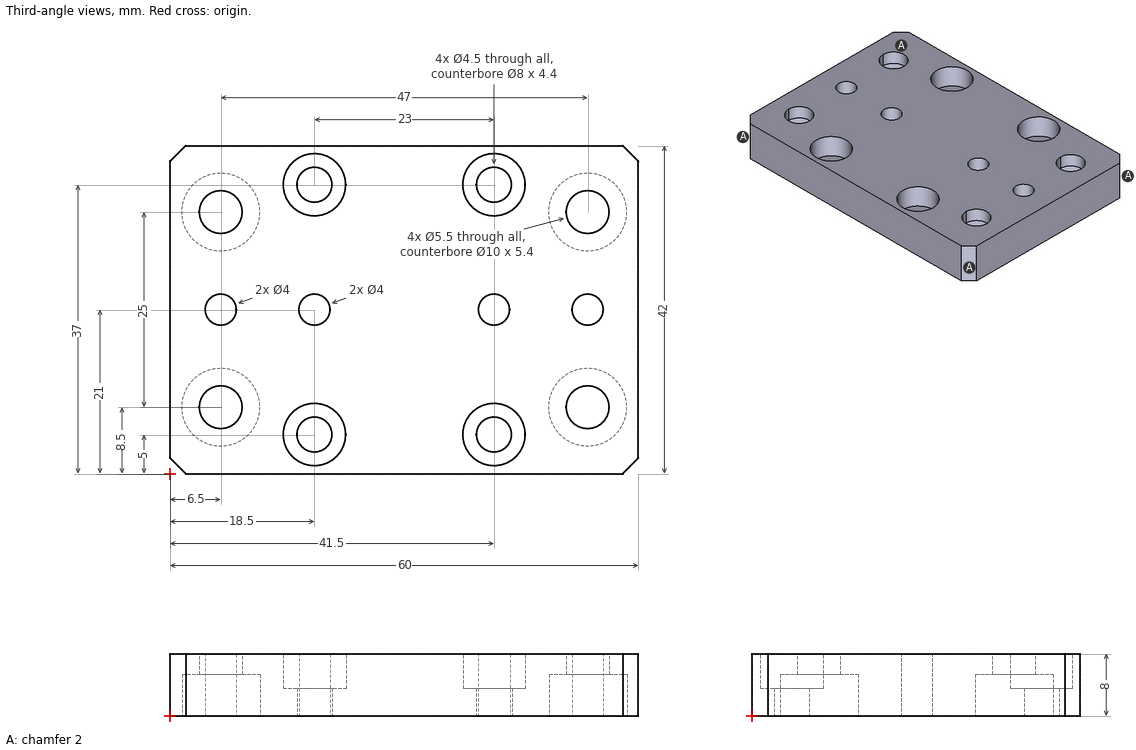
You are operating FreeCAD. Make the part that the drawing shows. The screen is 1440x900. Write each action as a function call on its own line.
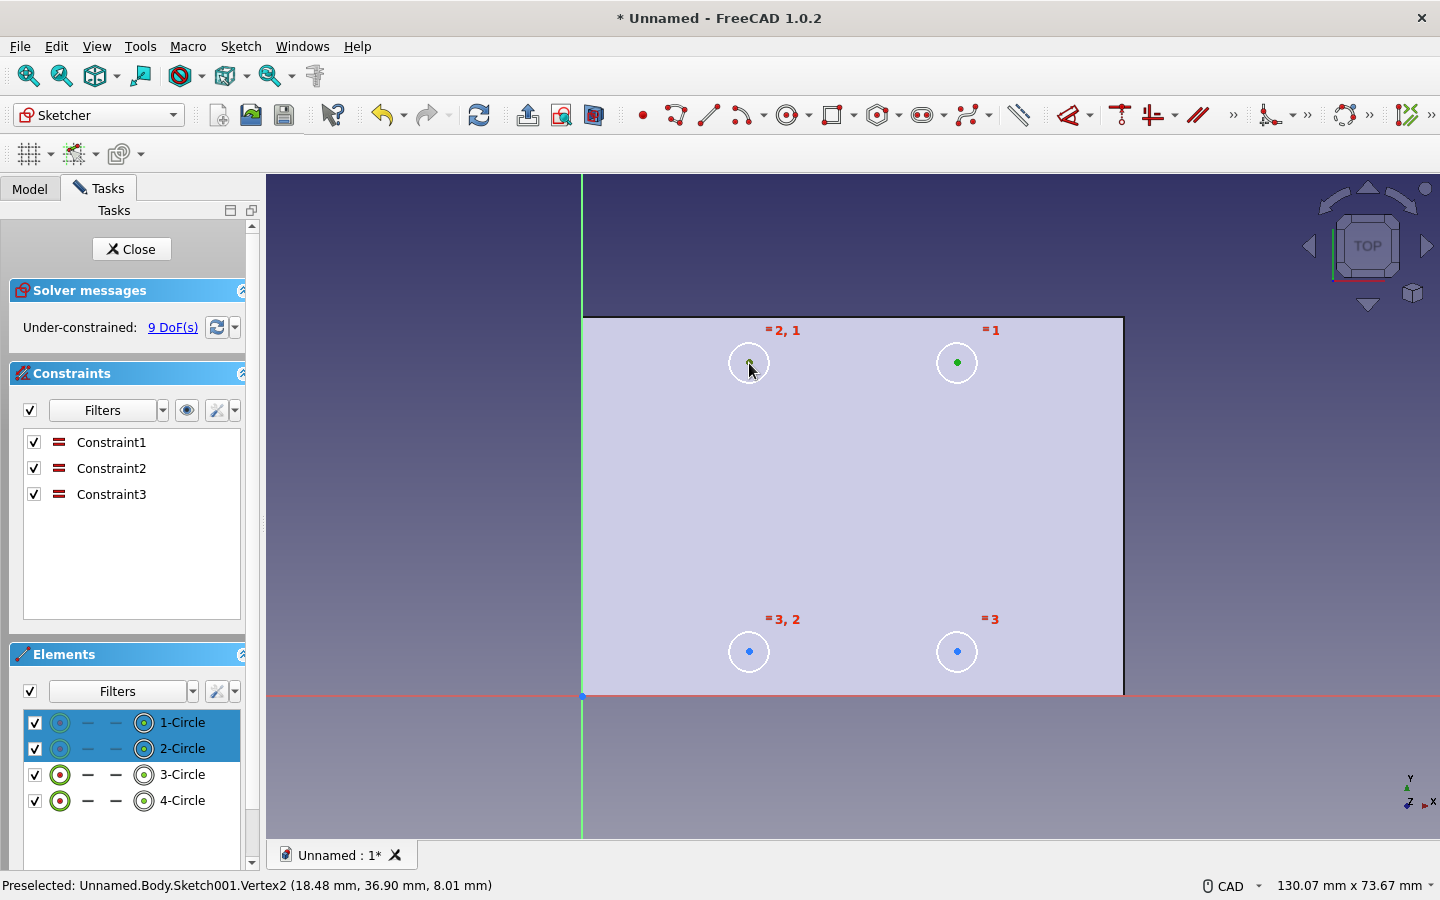
click(1174, 116)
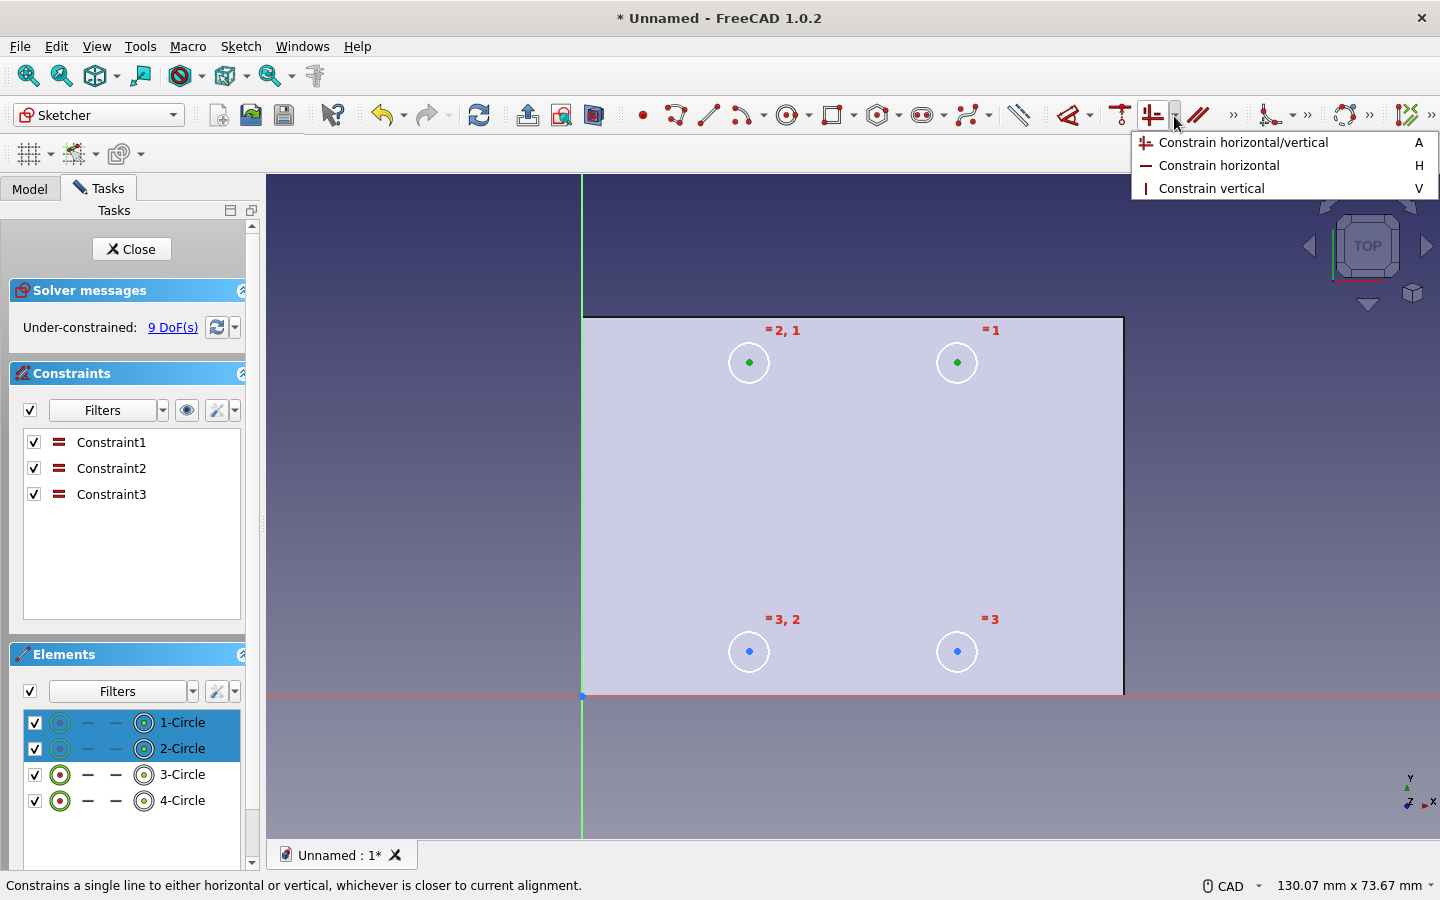
click(1285, 166)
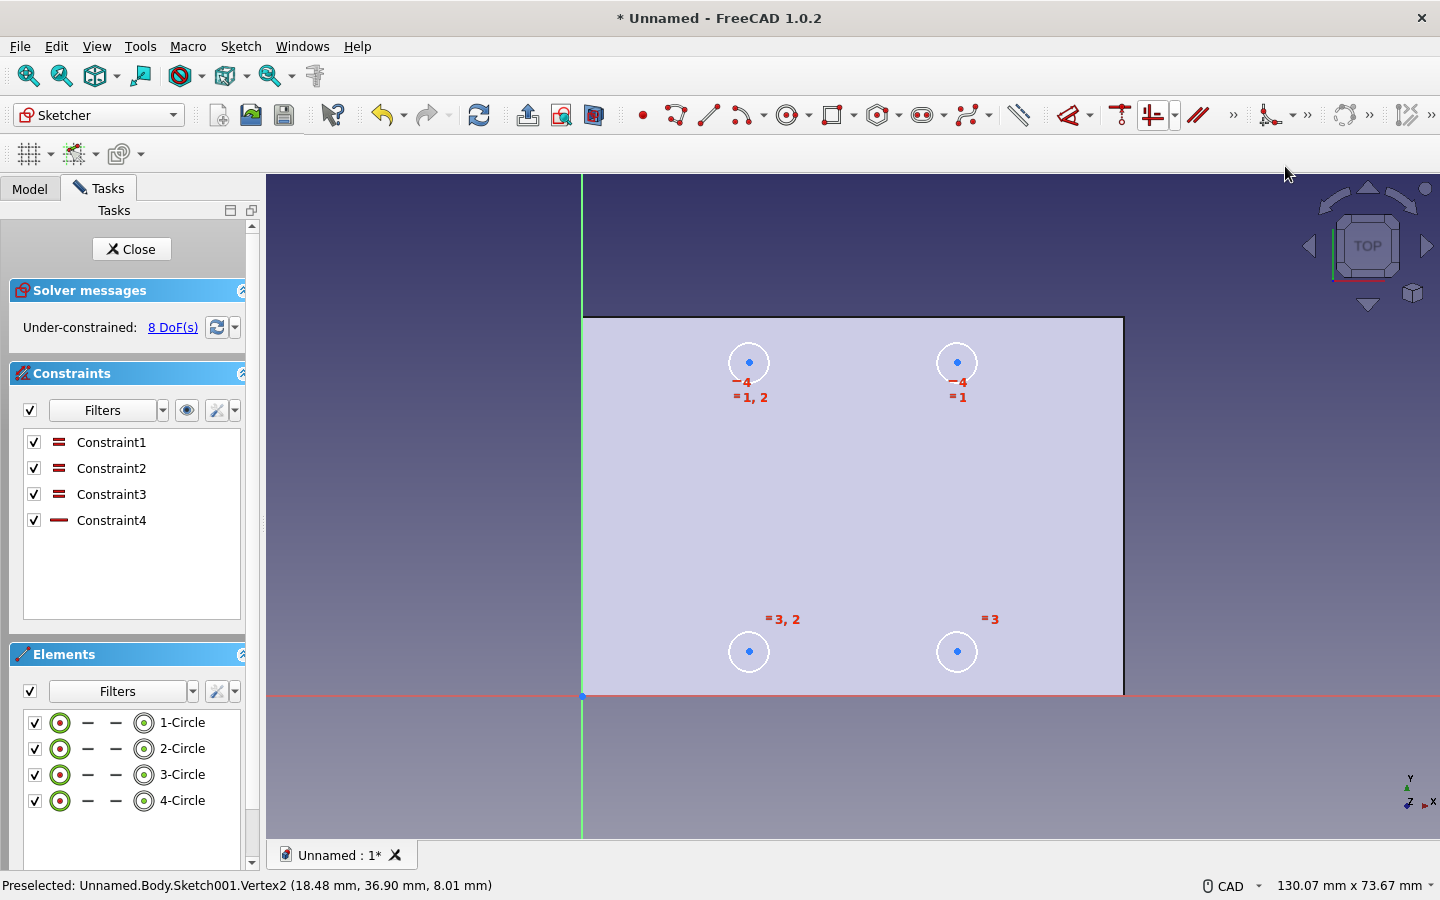
click(749, 363)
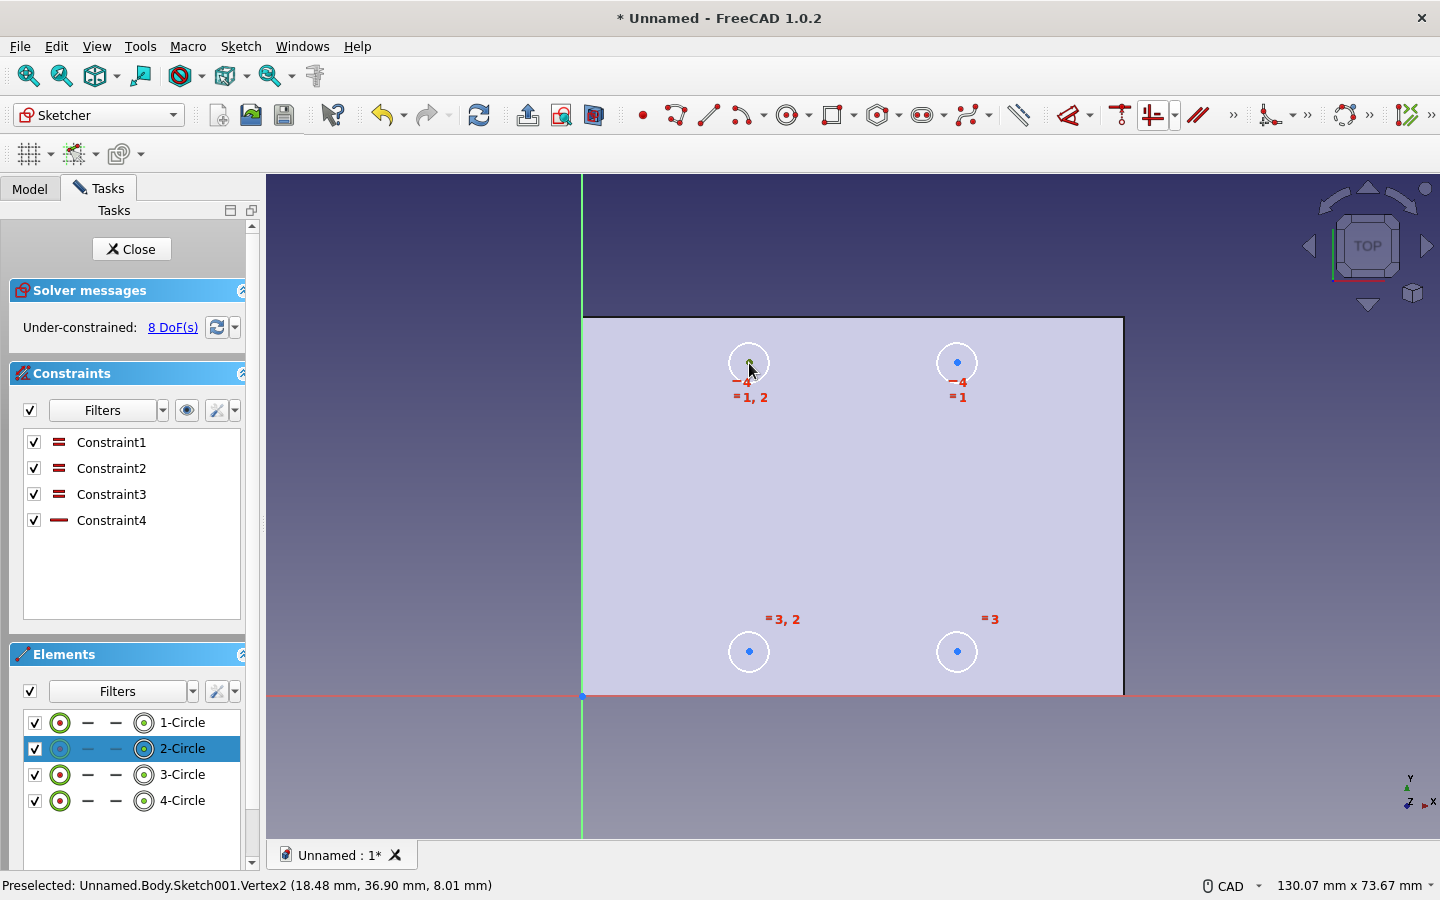
click(749, 652)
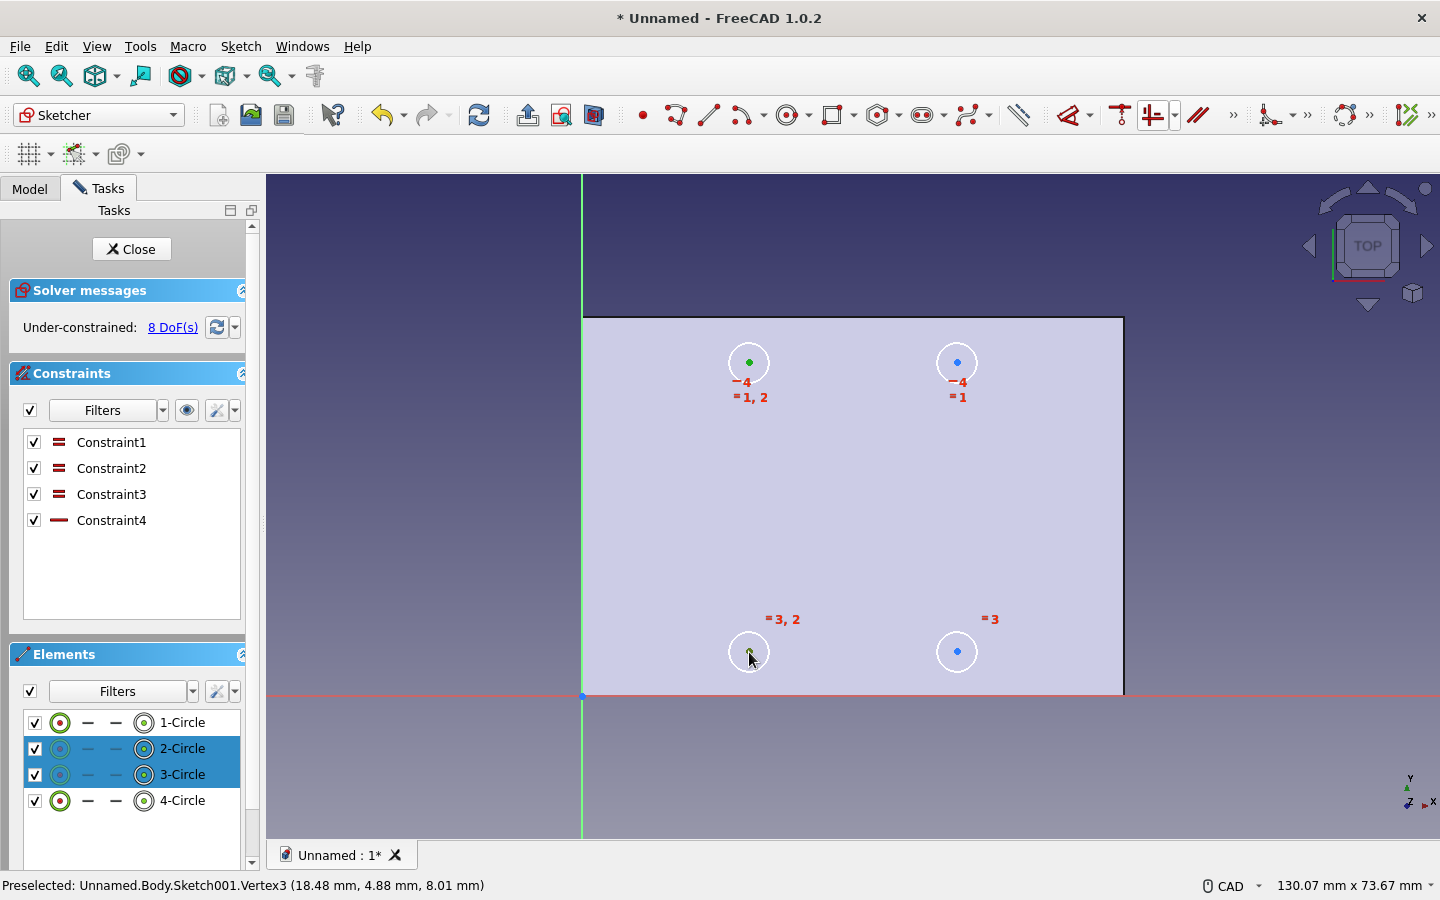
key(v)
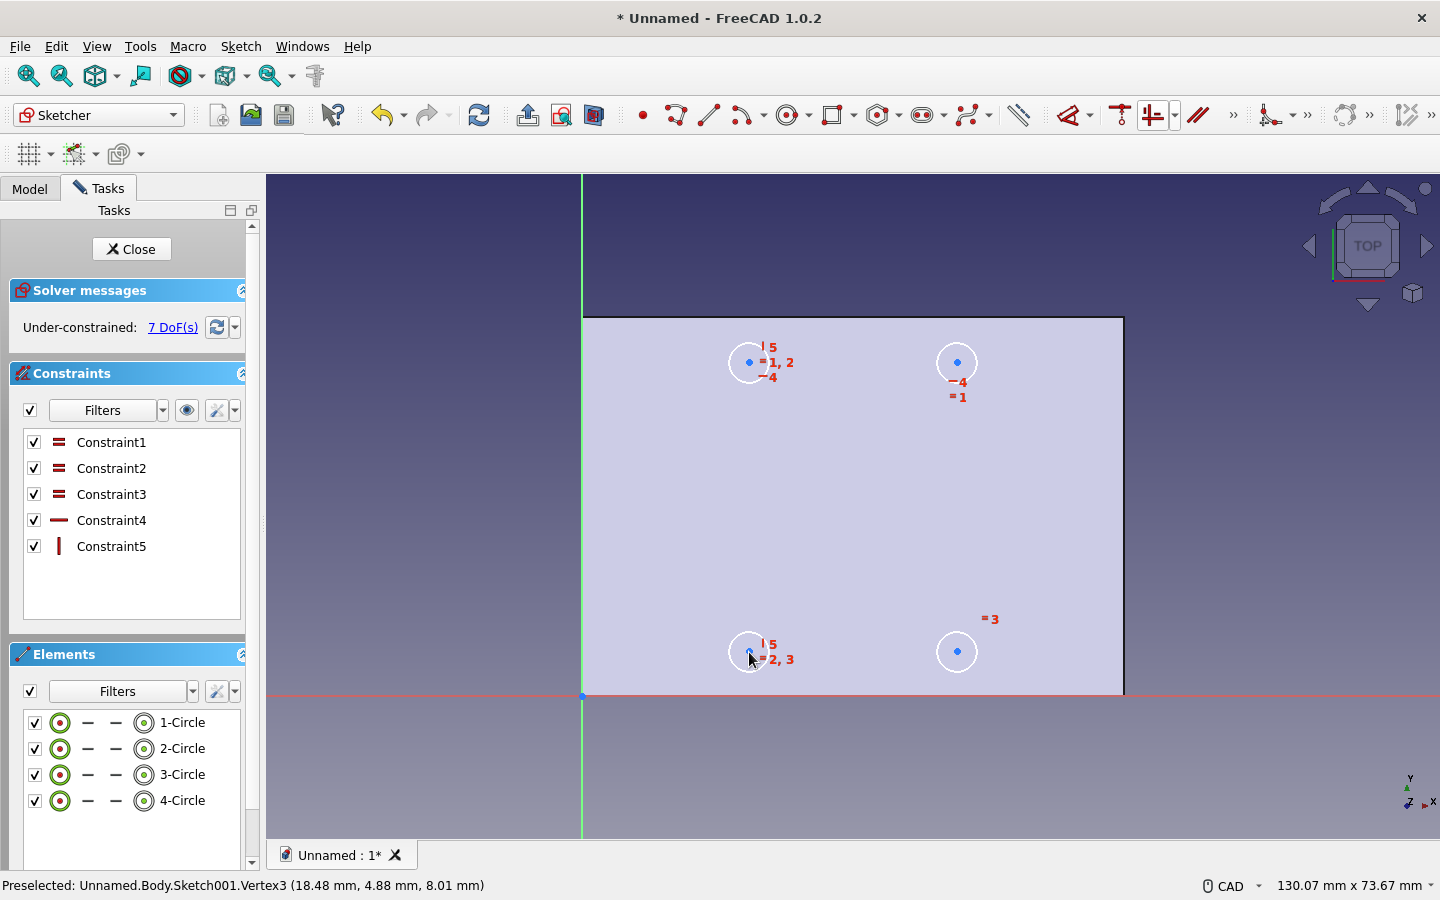
click(957, 363)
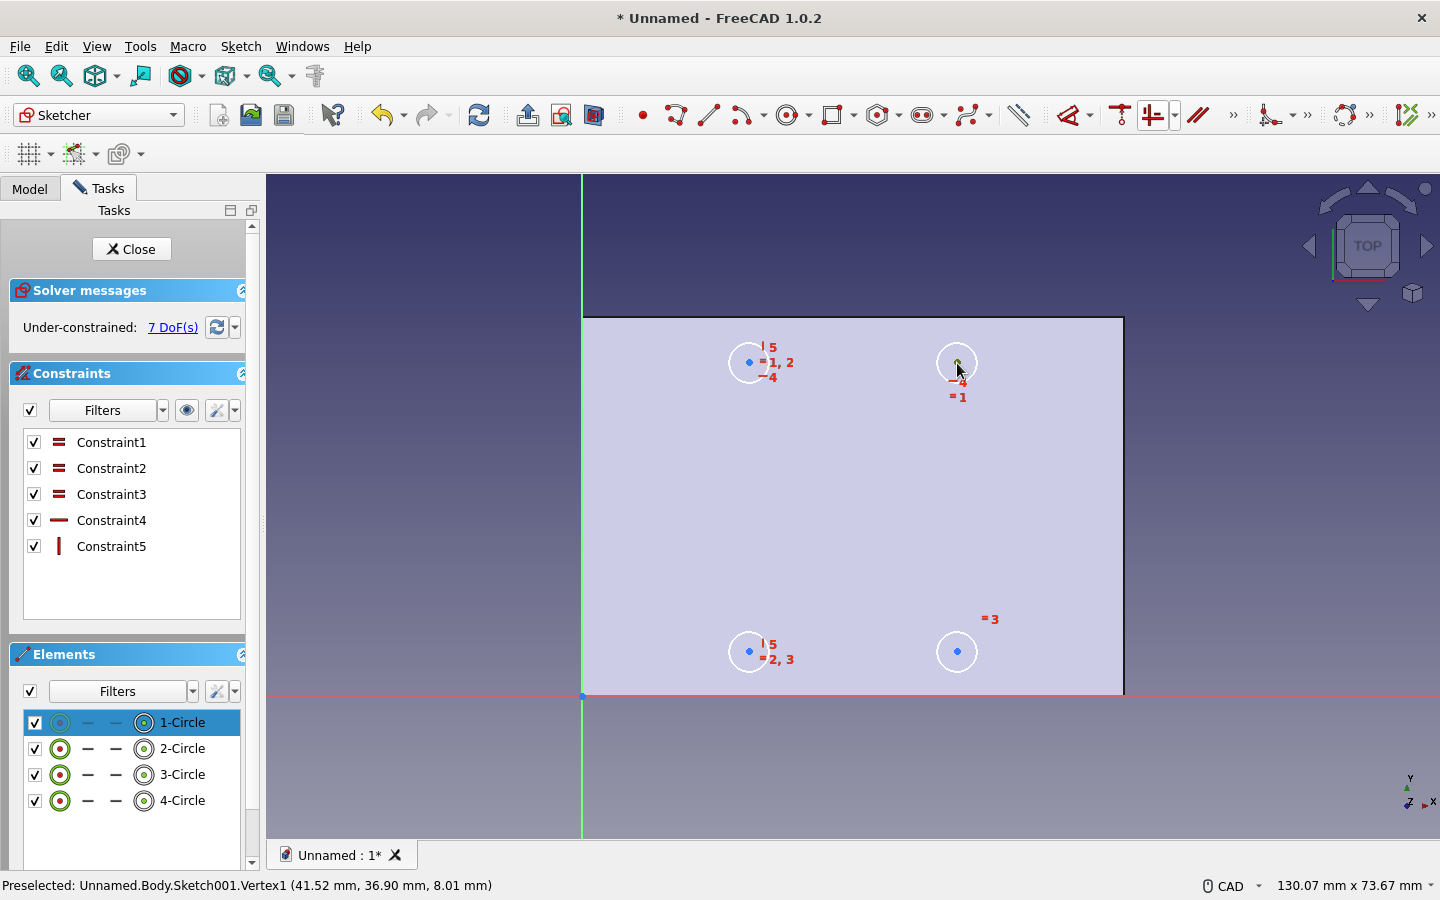
click(957, 652)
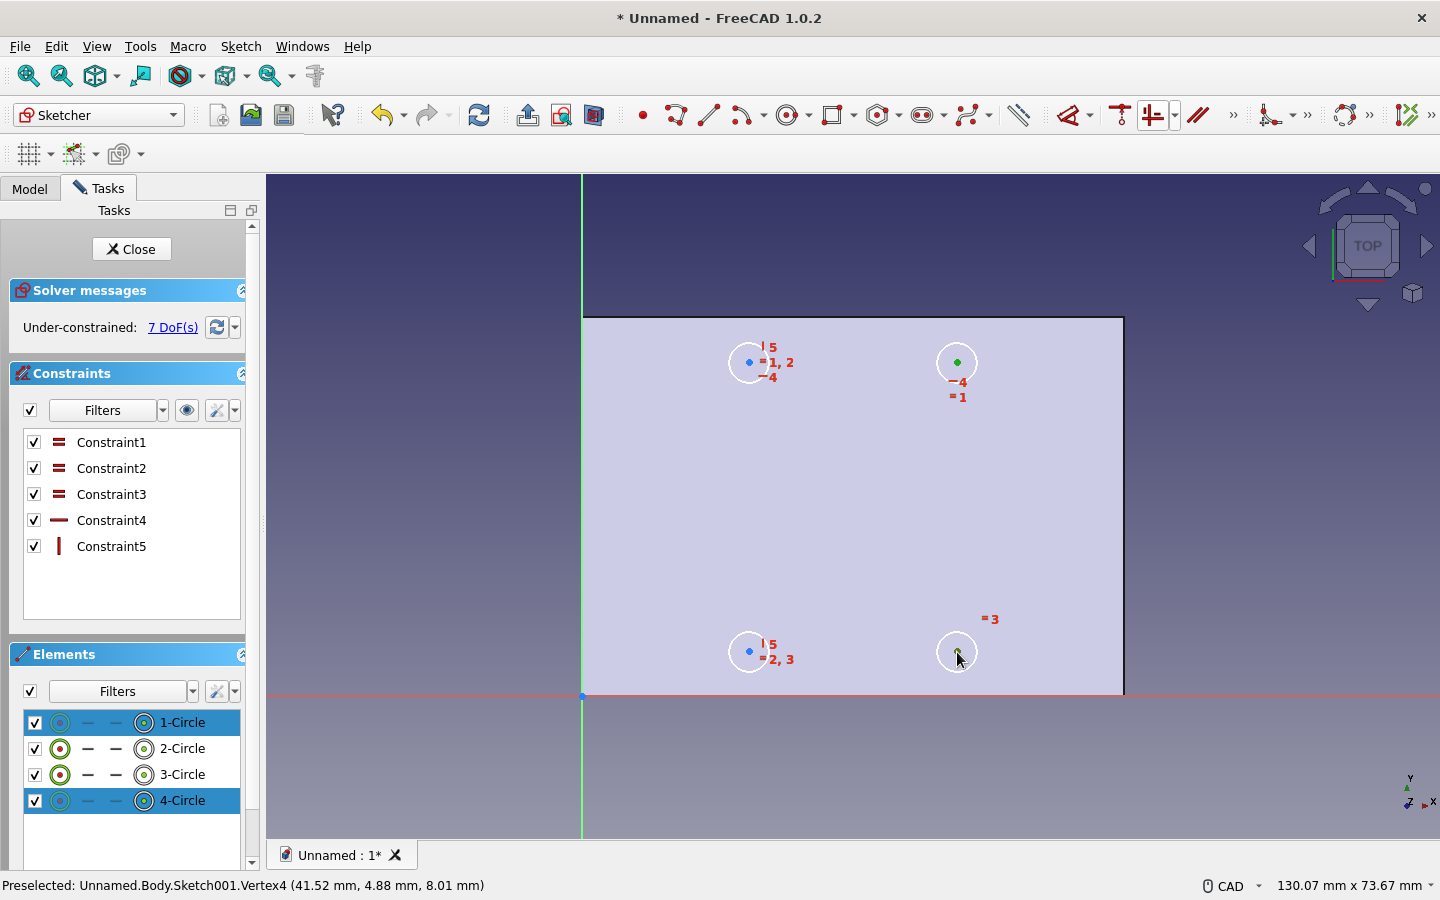
key(v)